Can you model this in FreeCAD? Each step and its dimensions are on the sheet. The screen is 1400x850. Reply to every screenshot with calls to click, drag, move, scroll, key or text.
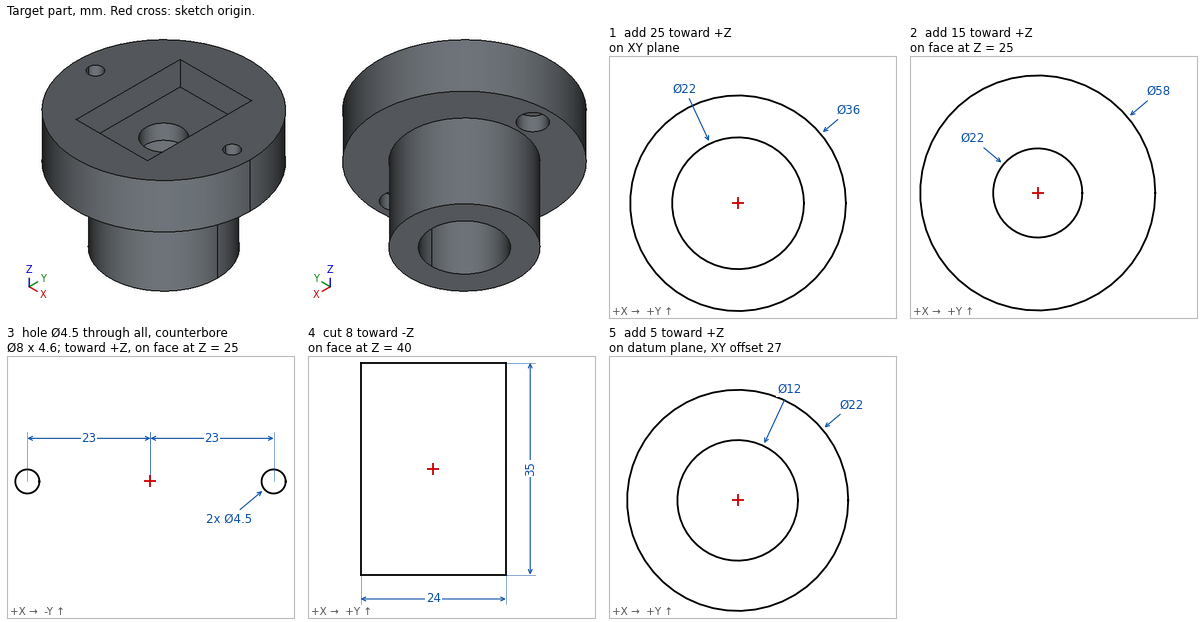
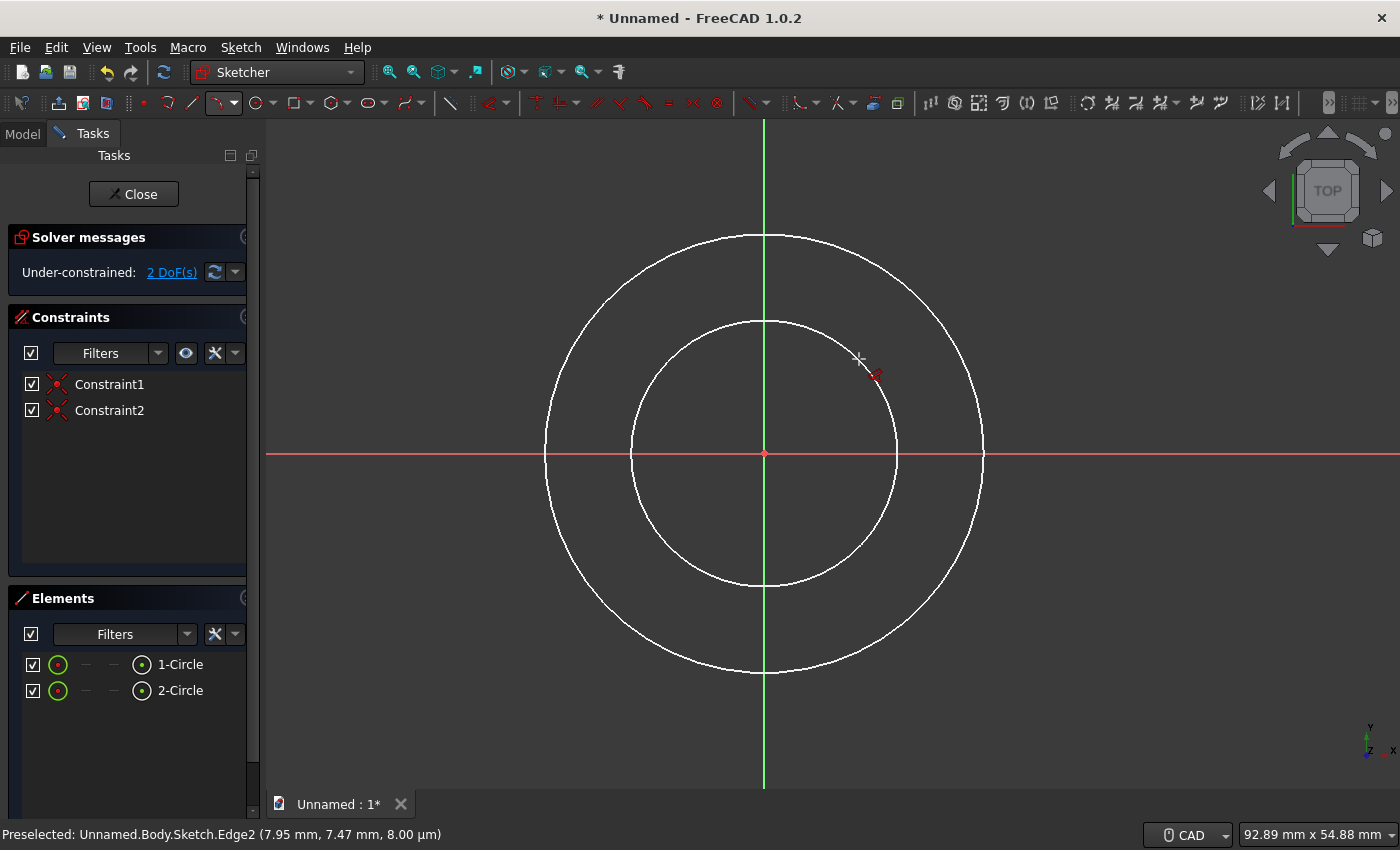
click(919, 298)
click(942, 275)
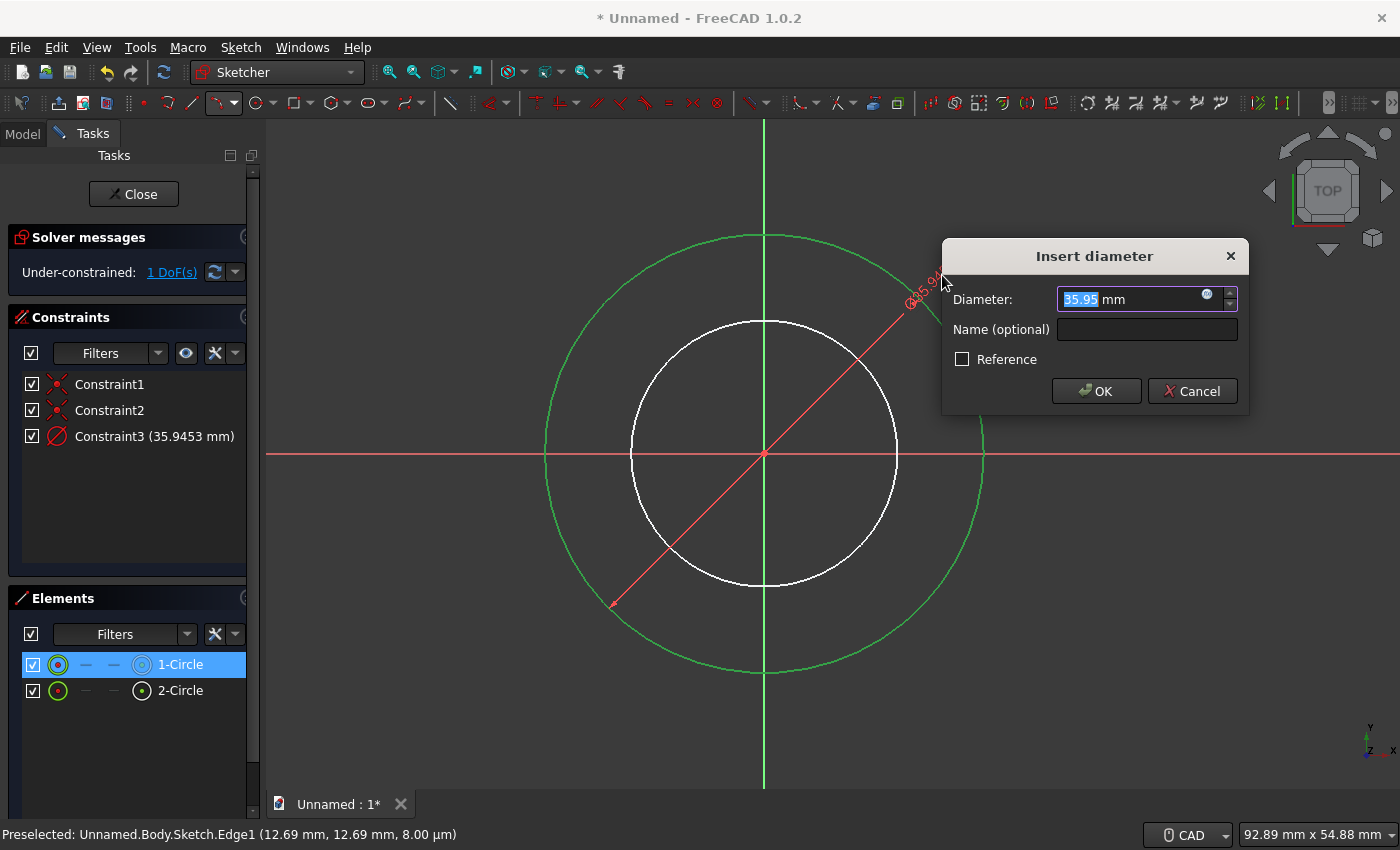
text(36)
key(Return)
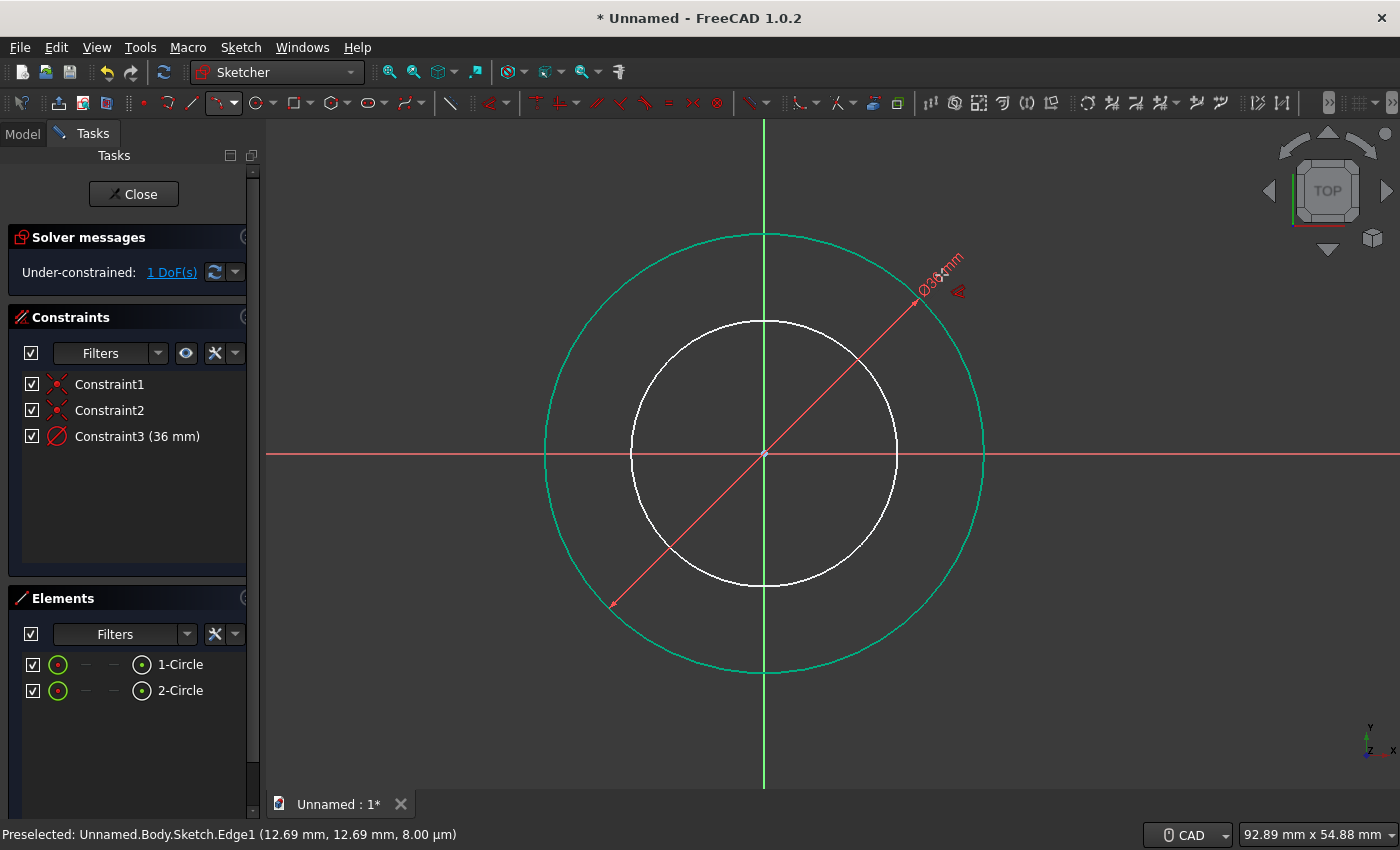
click(858, 359)
click(881, 336)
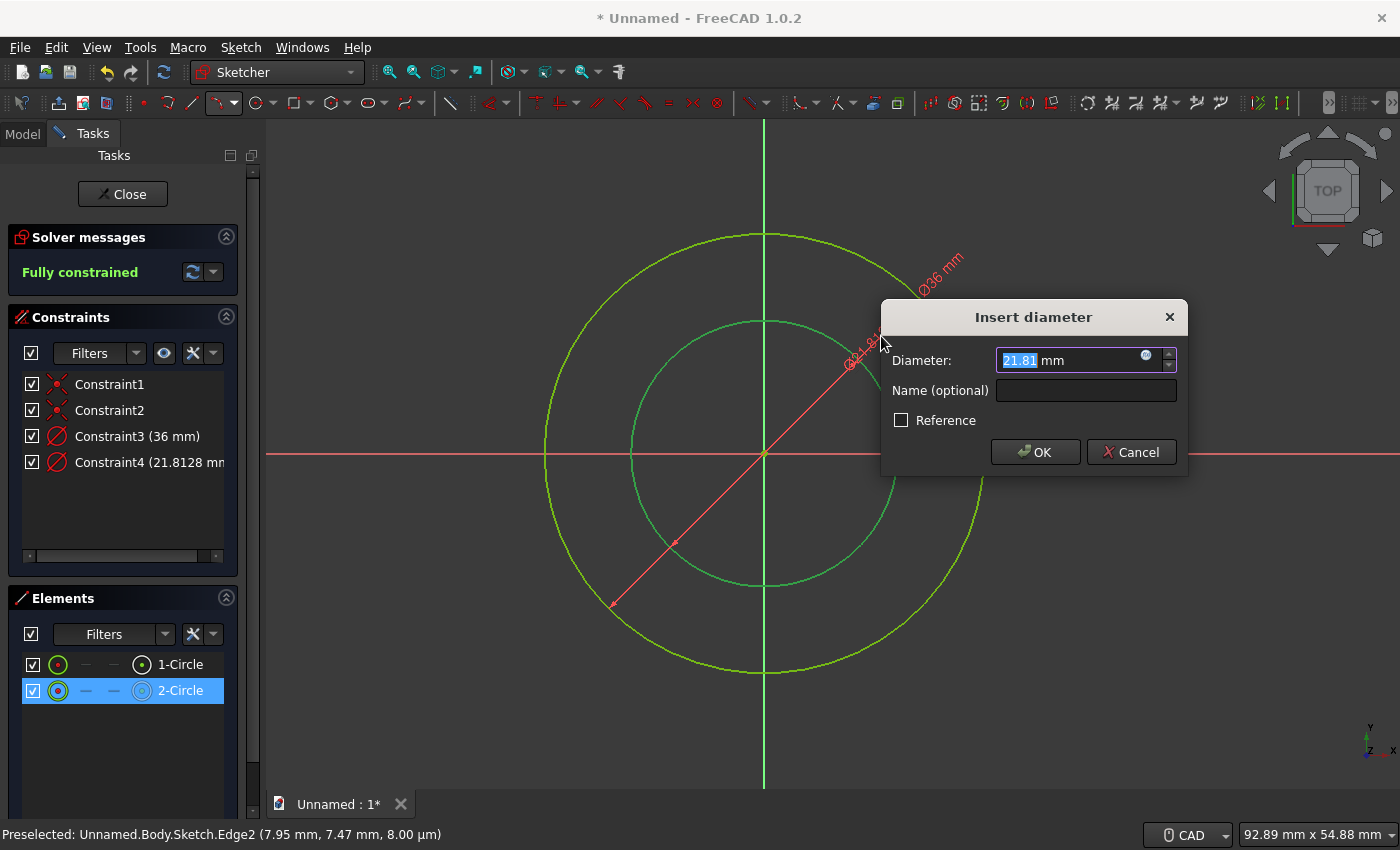
text(22)
key(Return)
key(Escape)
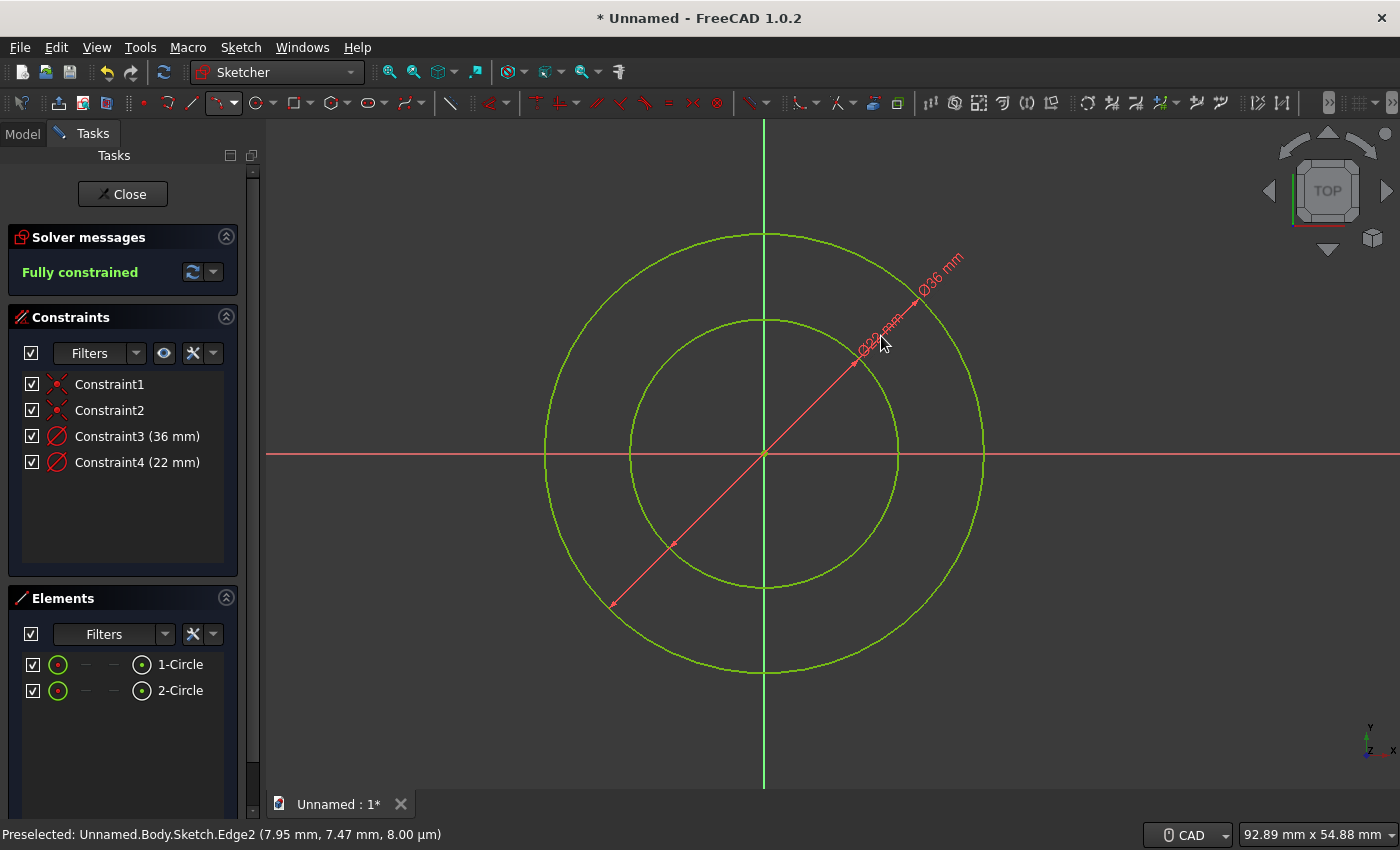
click(123, 194)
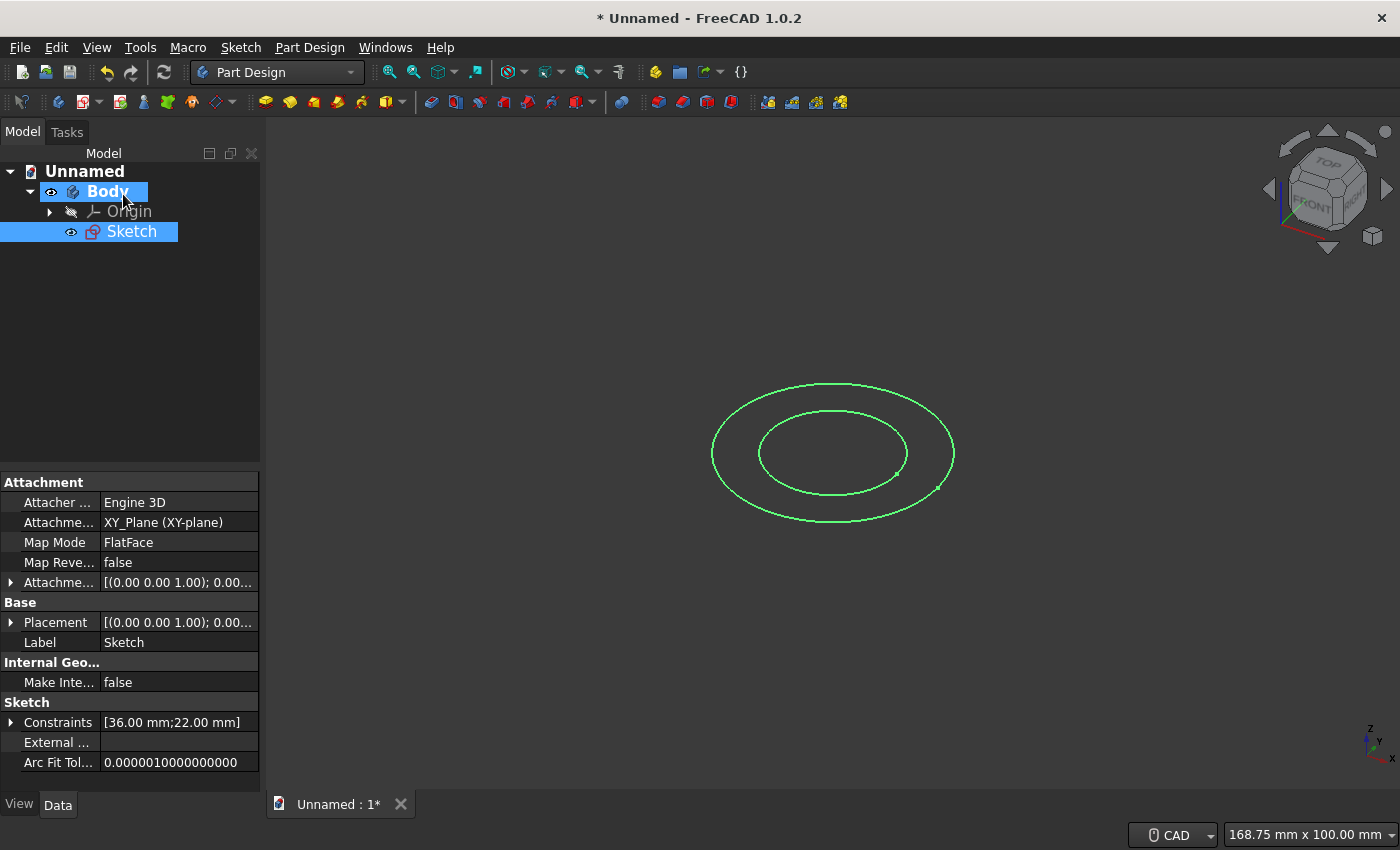
click(266, 102)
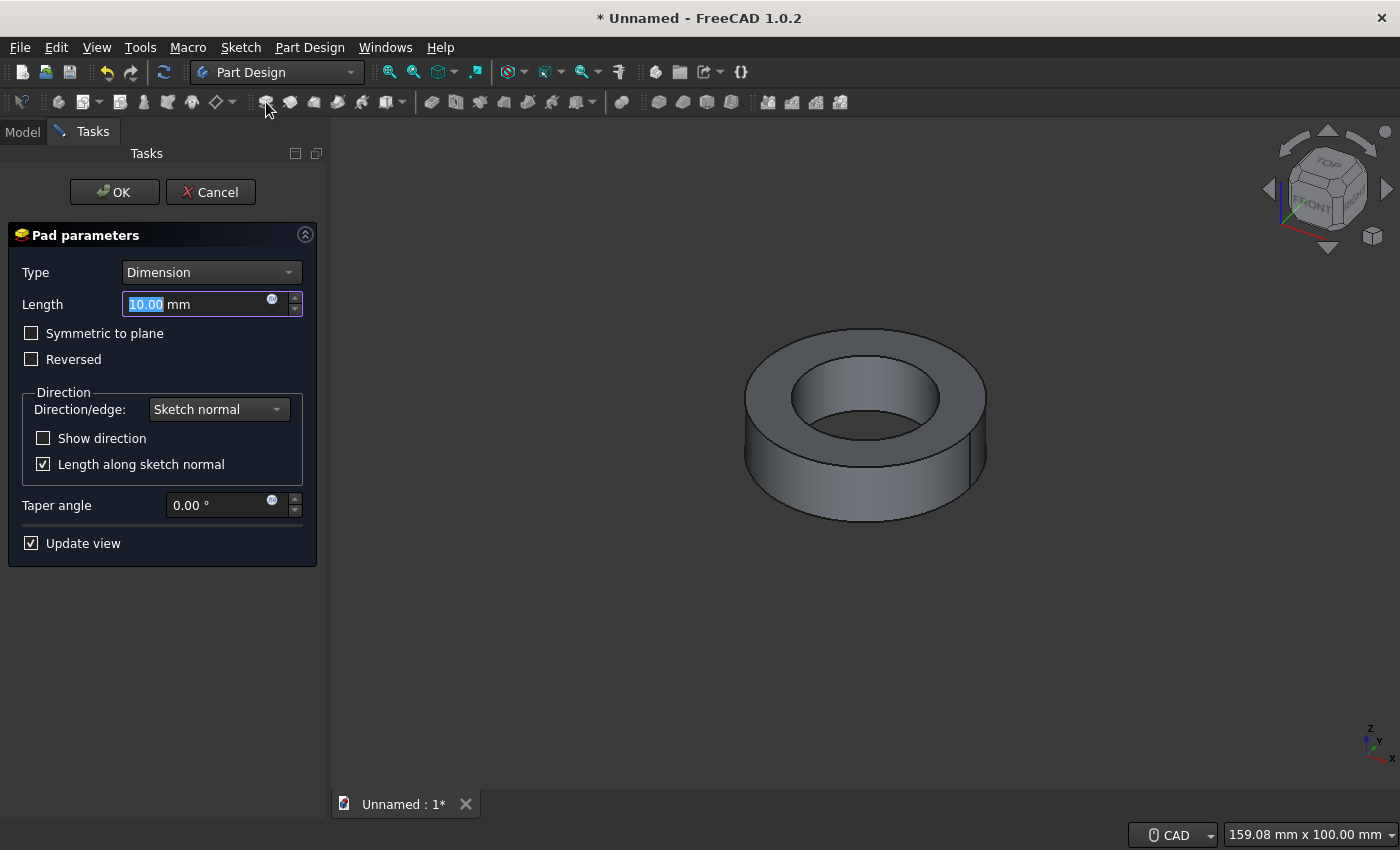
text(25)
key(Tab)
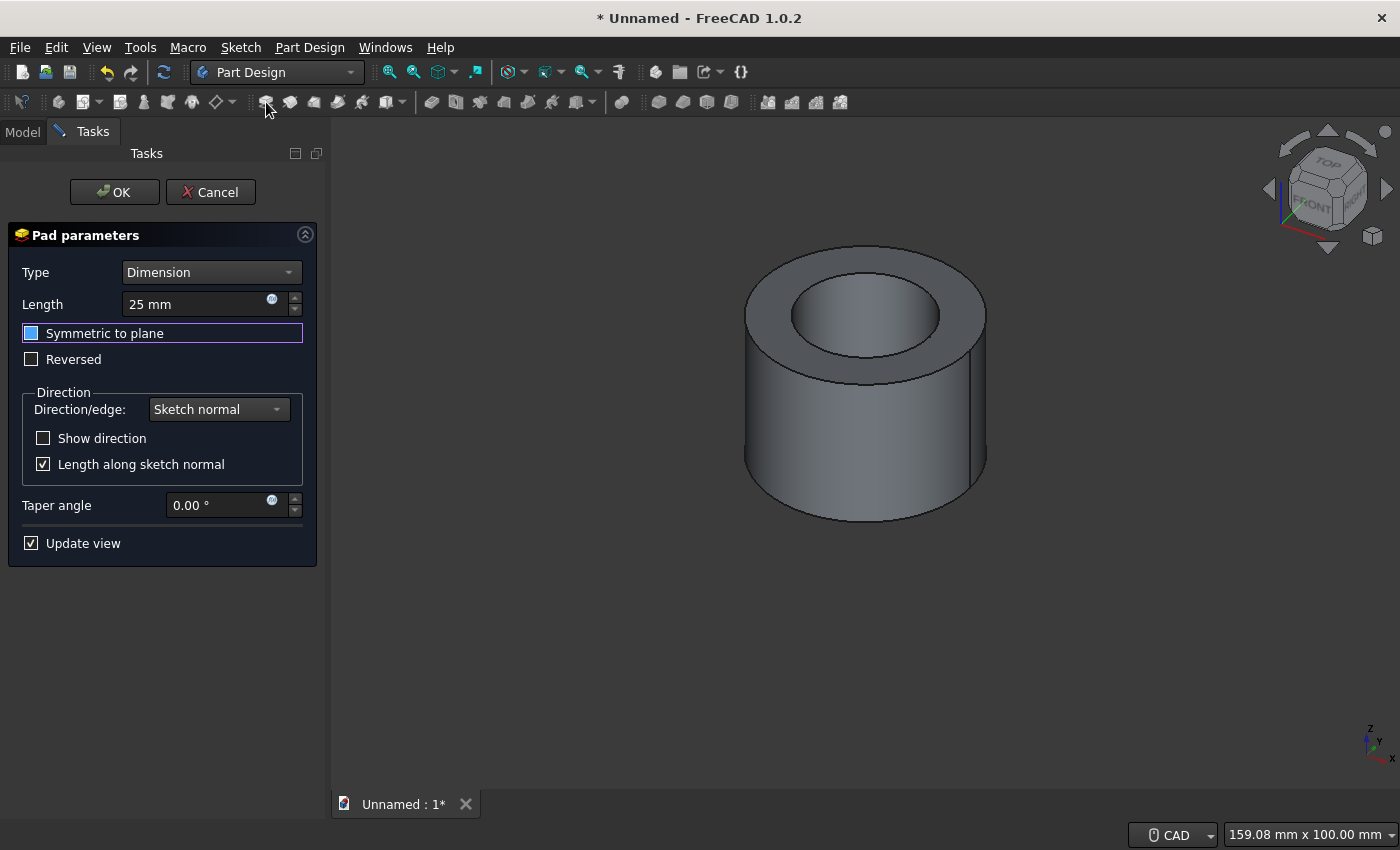
click(115, 192)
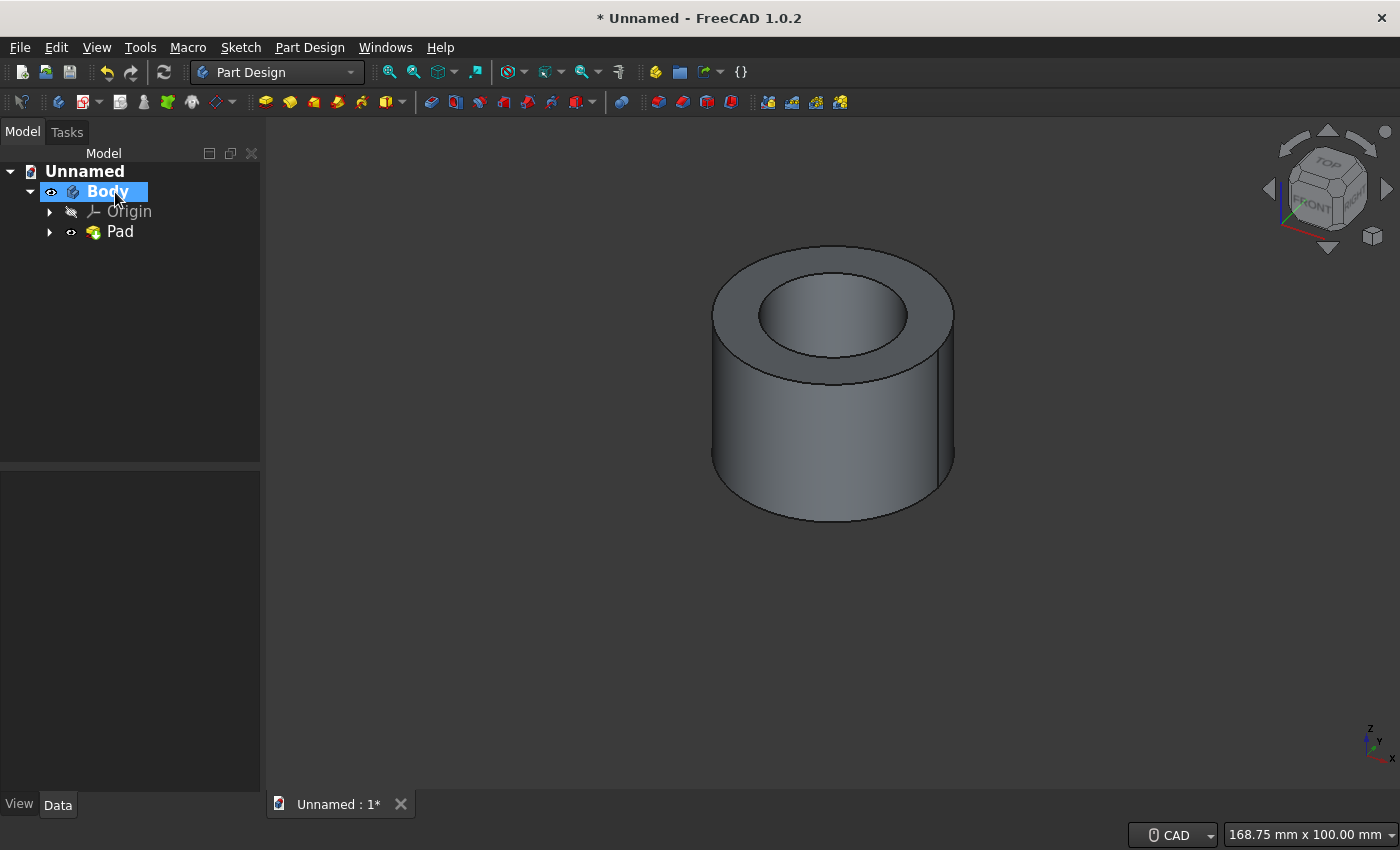
click(739, 329)